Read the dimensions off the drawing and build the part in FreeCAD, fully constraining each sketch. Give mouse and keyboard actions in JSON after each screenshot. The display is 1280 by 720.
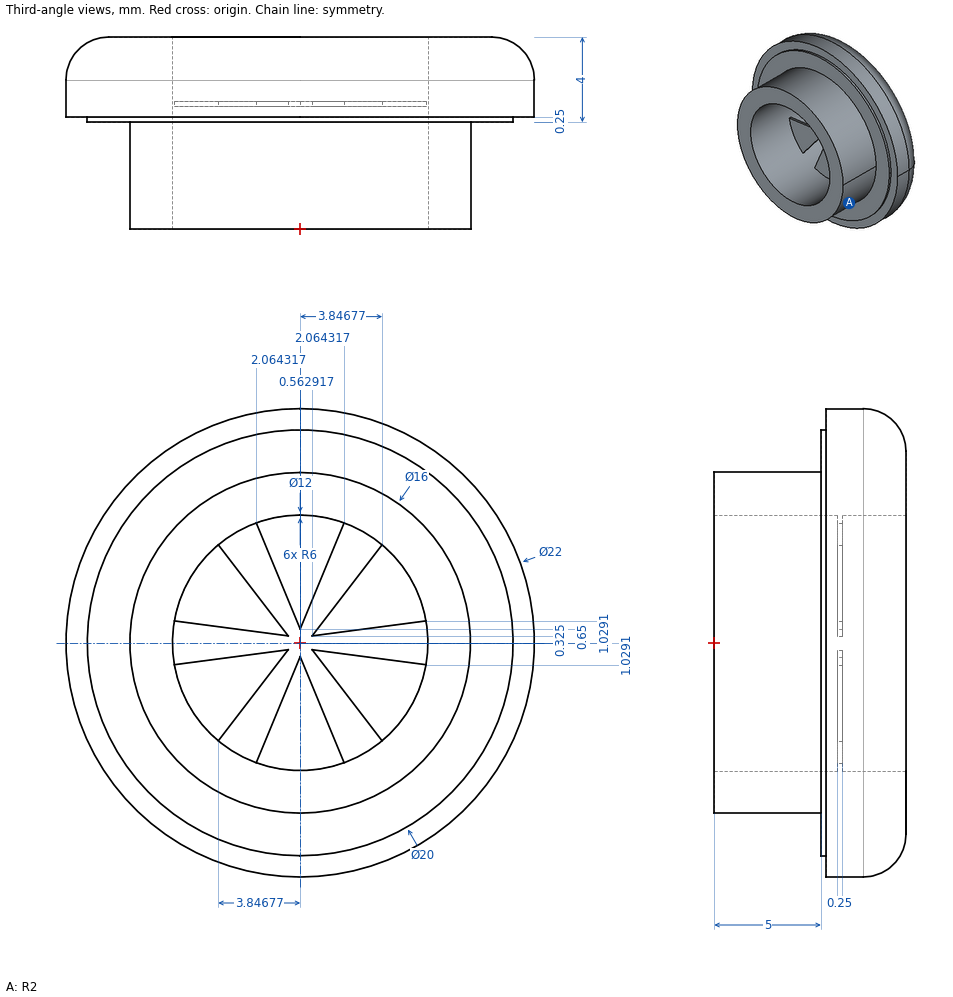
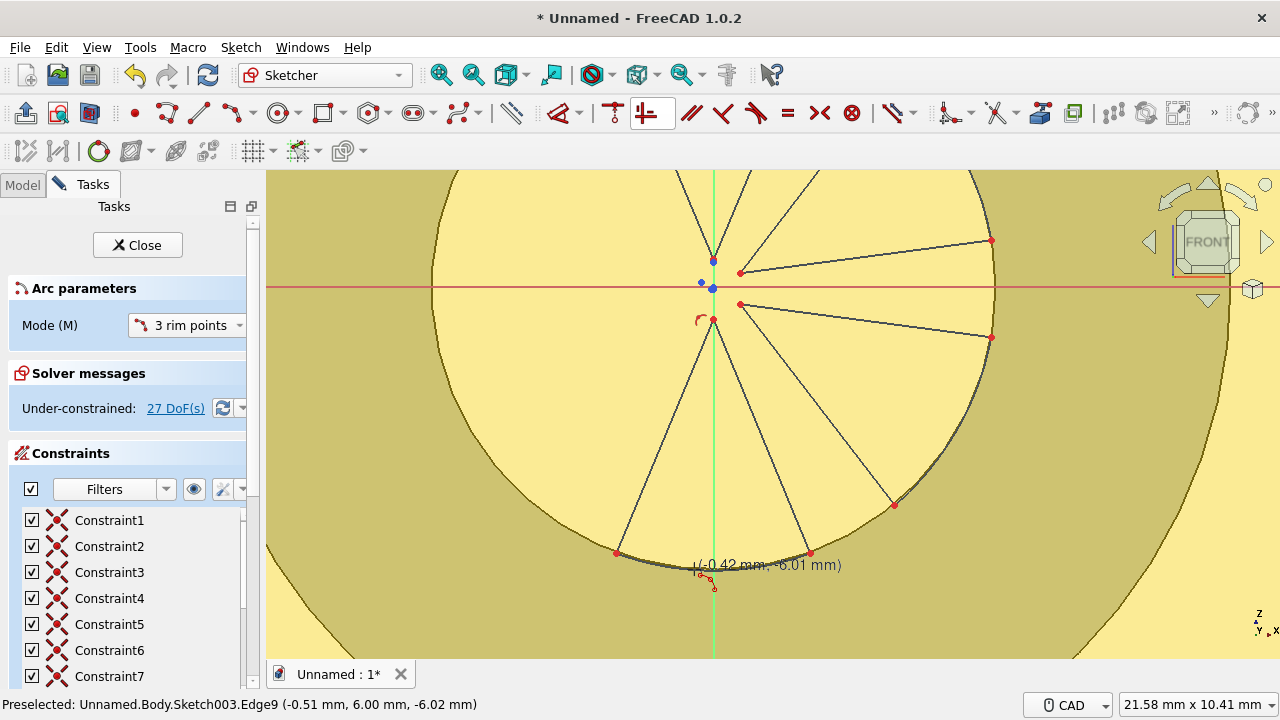
{"action": "left_click", "coordinate": [168, 114]}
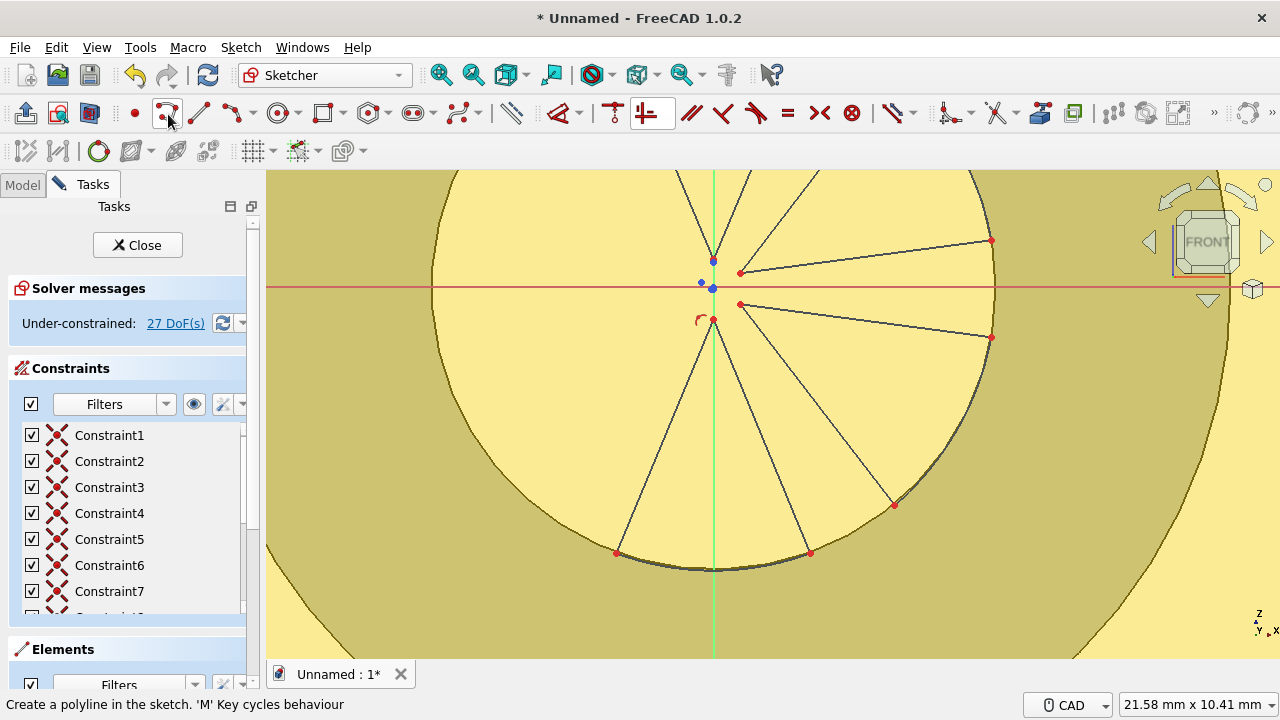
{"action": "left_click", "coordinate": [533, 504]}
{"action": "left_click", "coordinate": [687, 303]}
{"action": "left_click", "coordinate": [436, 336]}
{"action": "right_click", "coordinate": [436, 336]}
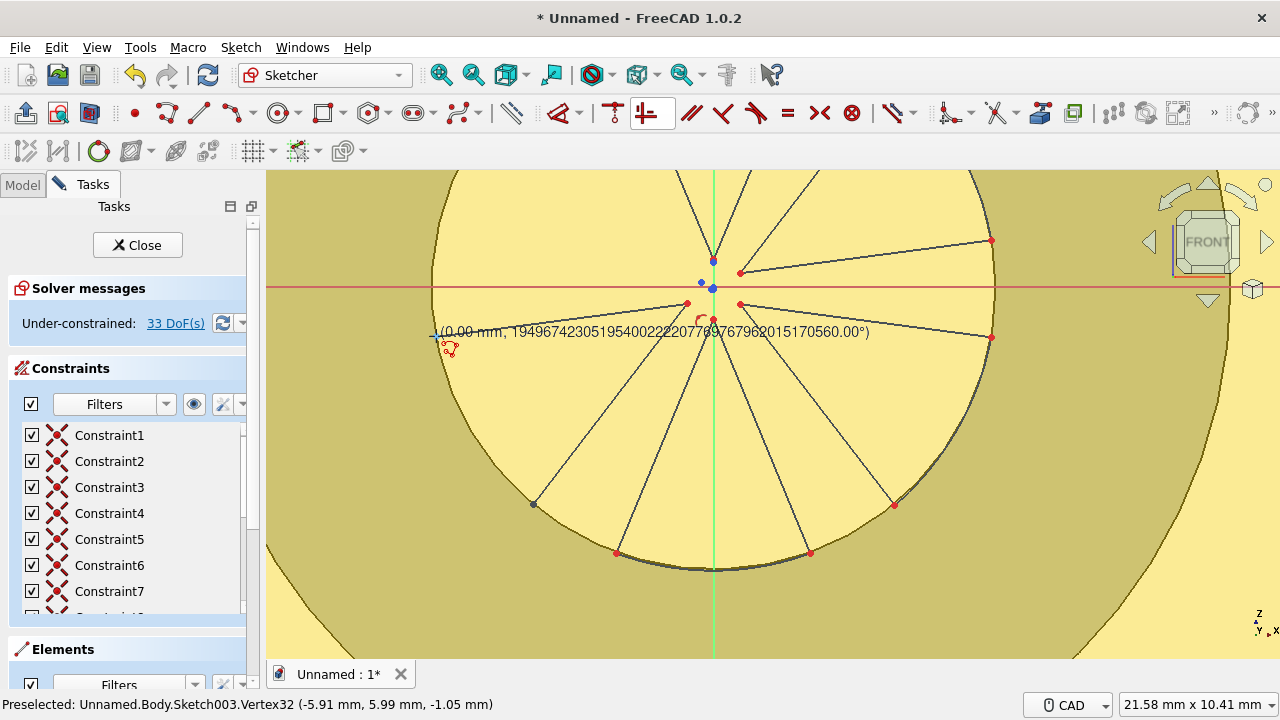
{"action": "key", "text": "g 3 a"}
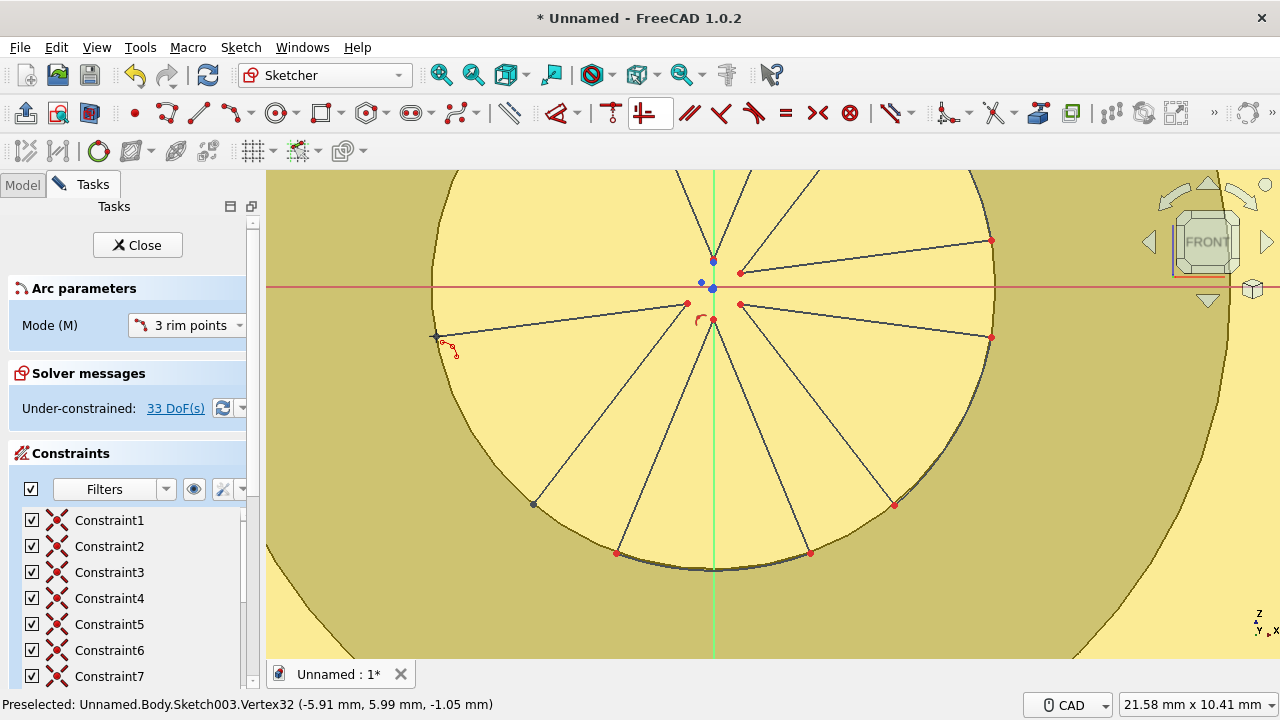
{"action": "left_click", "coordinate": [436, 337]}
{"action": "left_click", "coordinate": [533, 505]}
{"action": "left_click", "coordinate": [469, 428]}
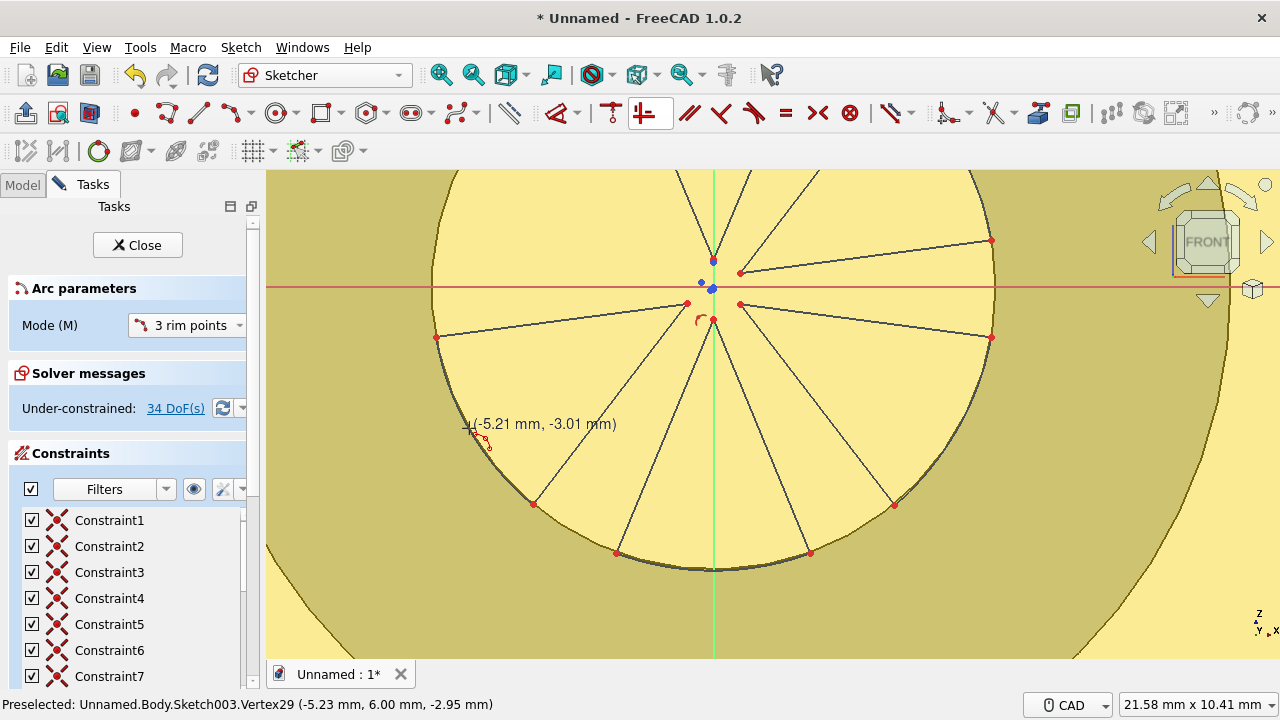
{"action": "key", "text": "g m"}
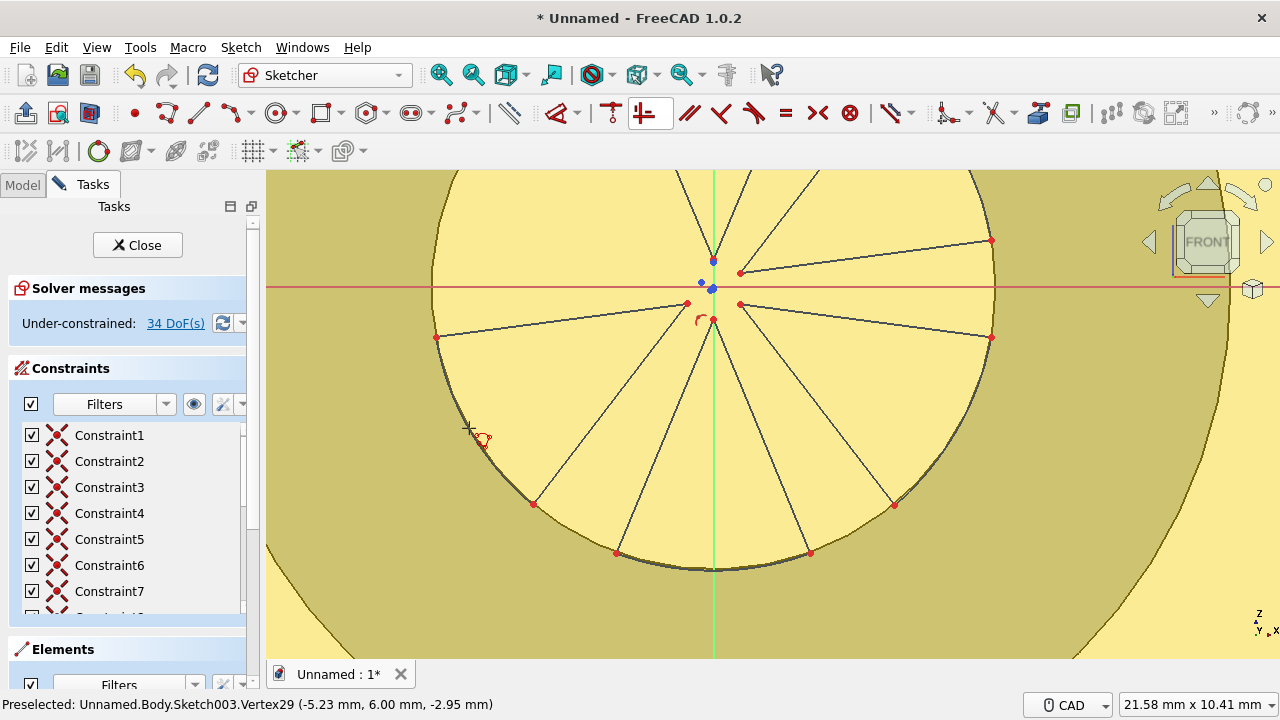
{"action": "left_click", "coordinate": [436, 239]}
{"action": "left_click", "coordinate": [687, 272]}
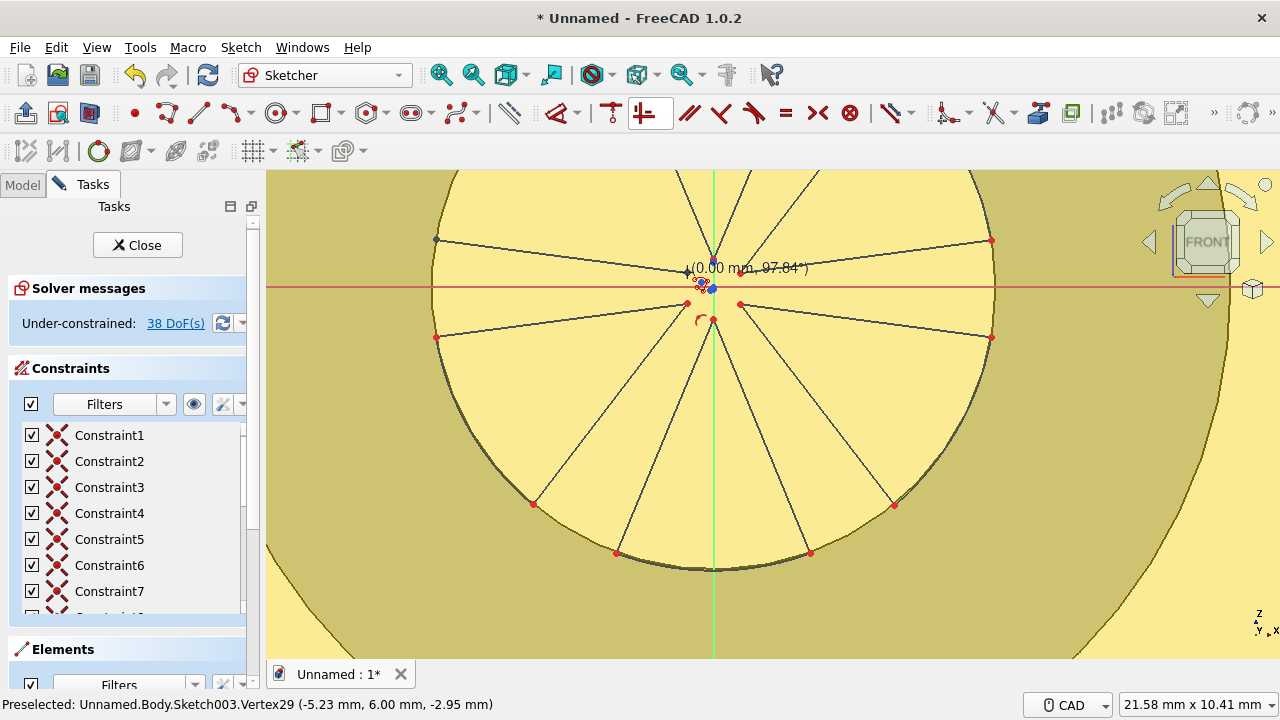
{"action": "scroll", "coordinate": [693, 569], "scroll_direction": "down", "scroll_amount": 3}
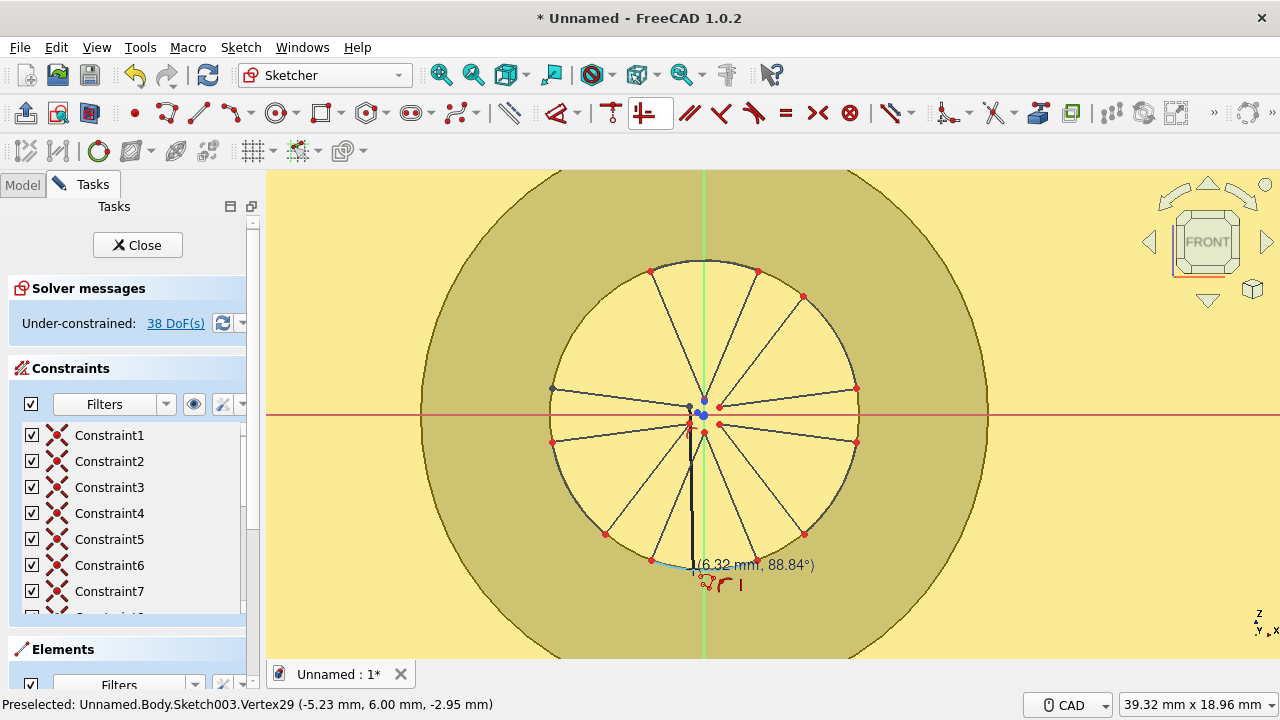
{"action": "left_click", "coordinate": [605, 296]}
{"action": "right_click", "coordinate": [605, 296]}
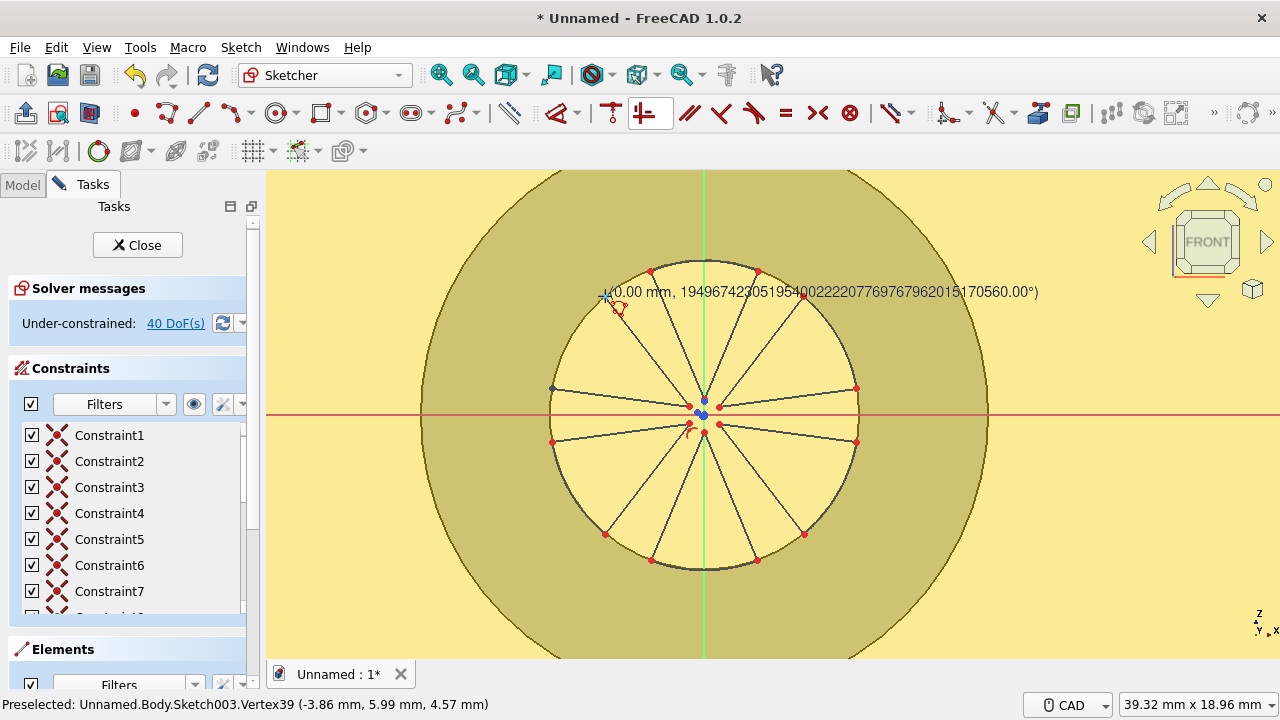
{"action": "key", "text": "g 3 a"}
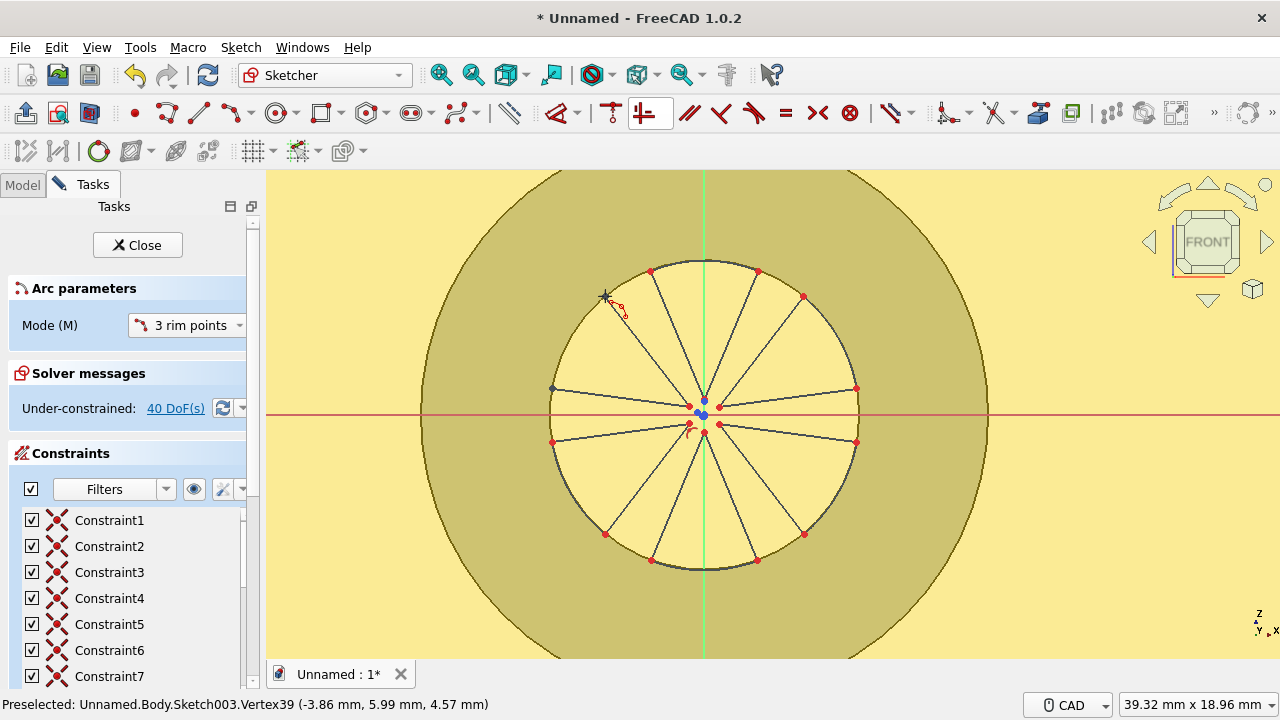
{"action": "left_click", "coordinate": [605, 297]}
{"action": "left_click", "coordinate": [552, 389]}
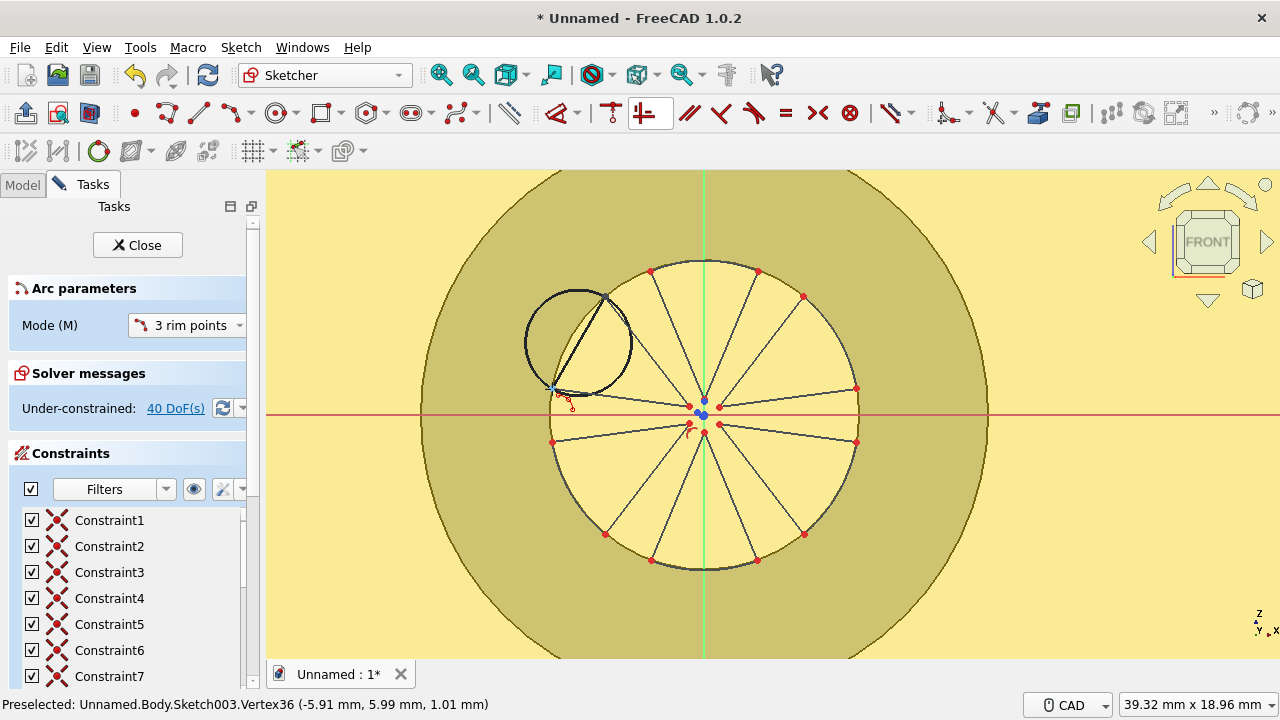
{"action": "scroll", "coordinate": [570, 338], "scroll_direction": "up", "scroll_amount": 3}